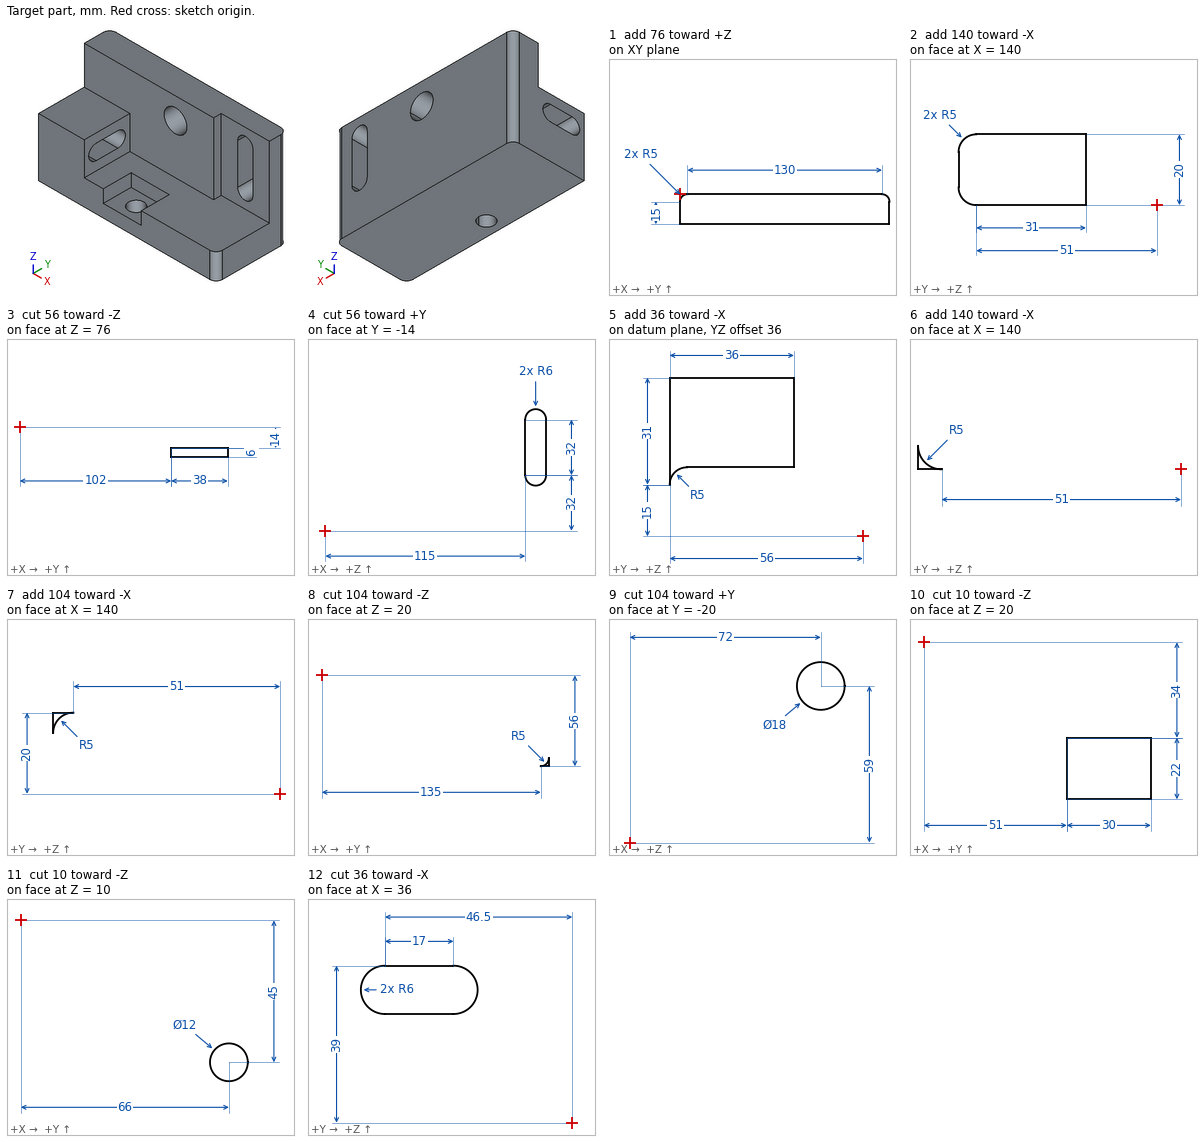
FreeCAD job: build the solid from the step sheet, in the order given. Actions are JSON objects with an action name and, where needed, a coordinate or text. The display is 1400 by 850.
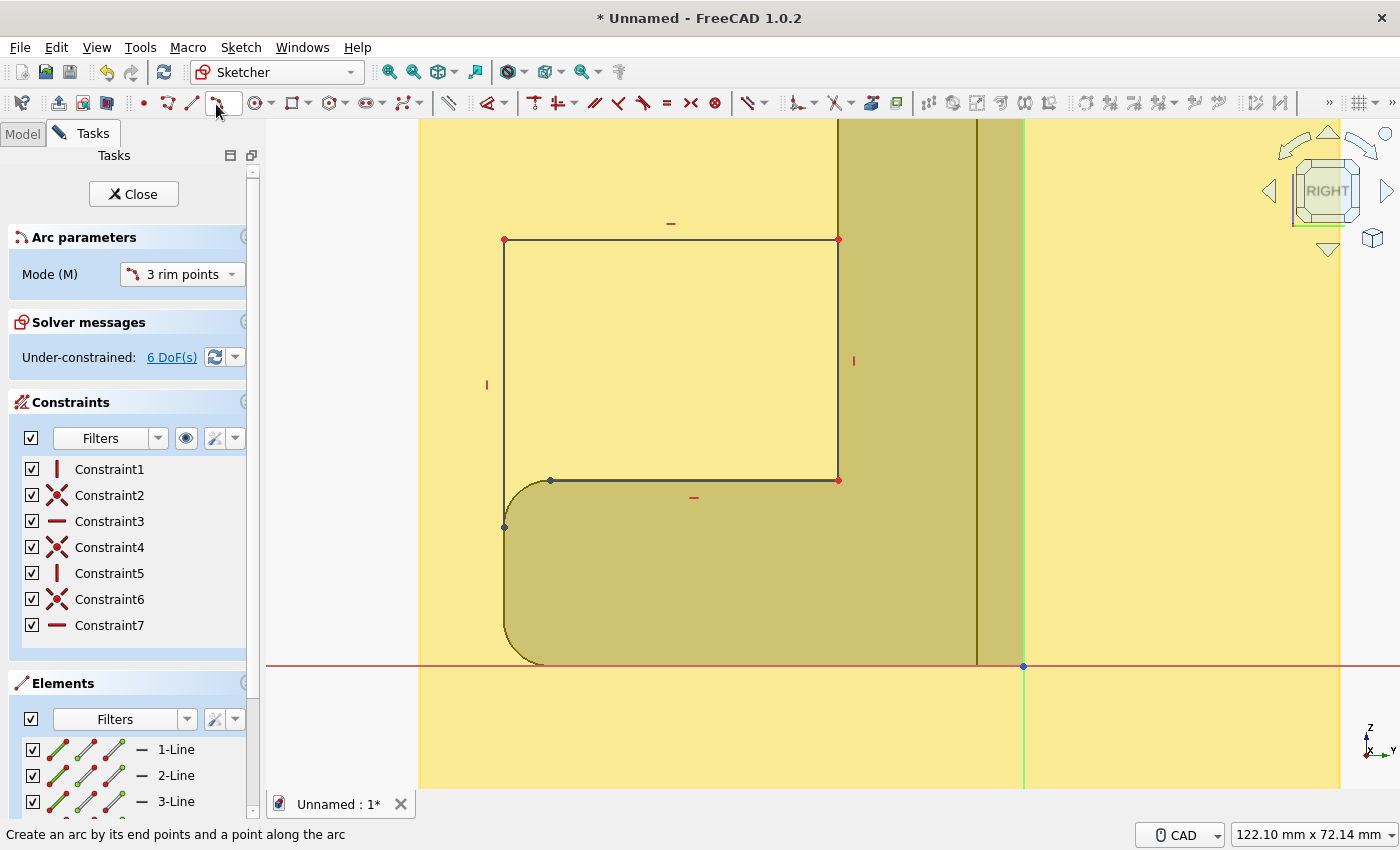
{"action": "left_click", "coordinate": [550, 481]}
{"action": "left_click", "coordinate": [504, 528]}
{"action": "left_click", "coordinate": [517, 494]}
{"action": "key", "text": "Escape"}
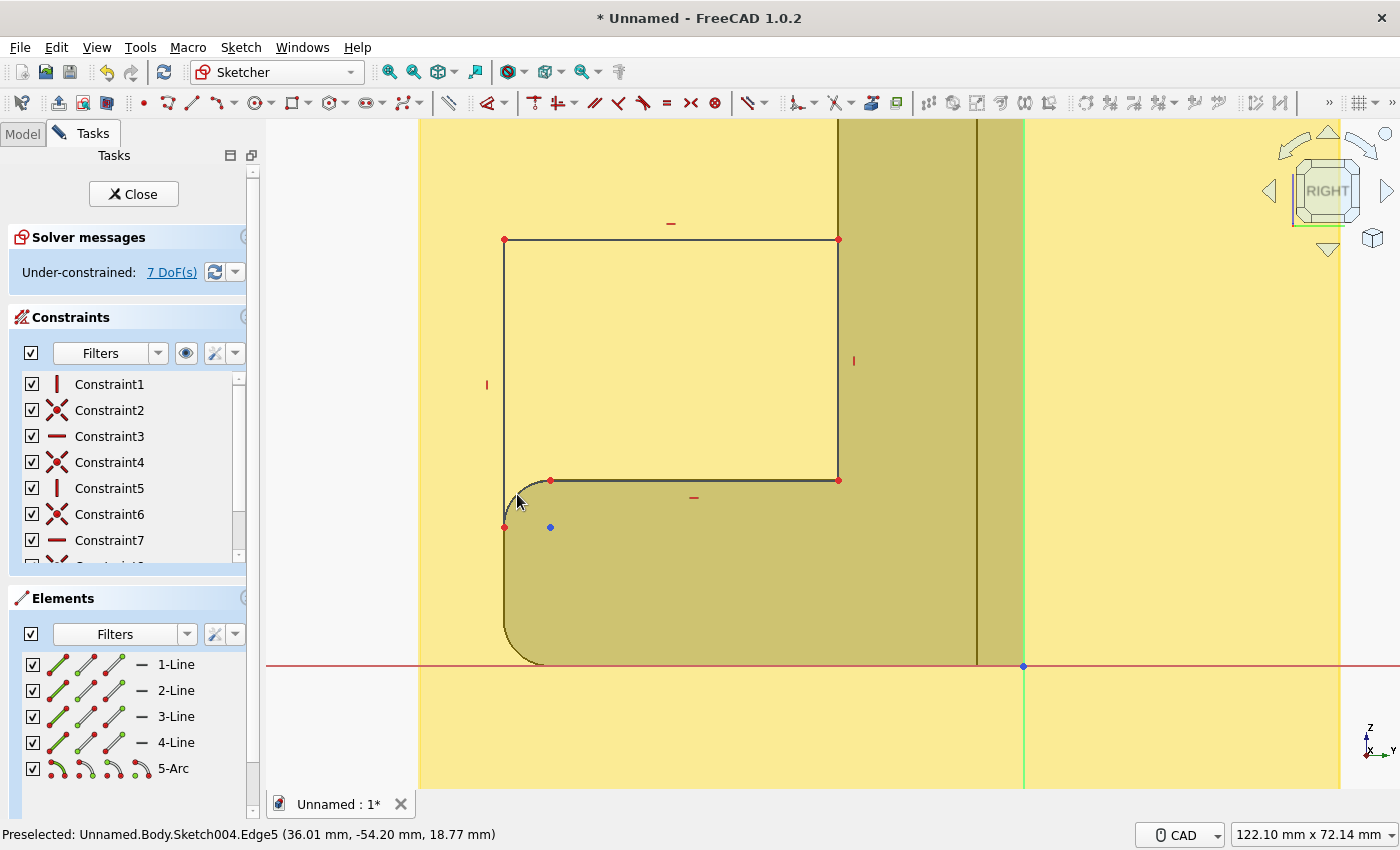
{"action": "left_click", "coordinate": [504, 442]}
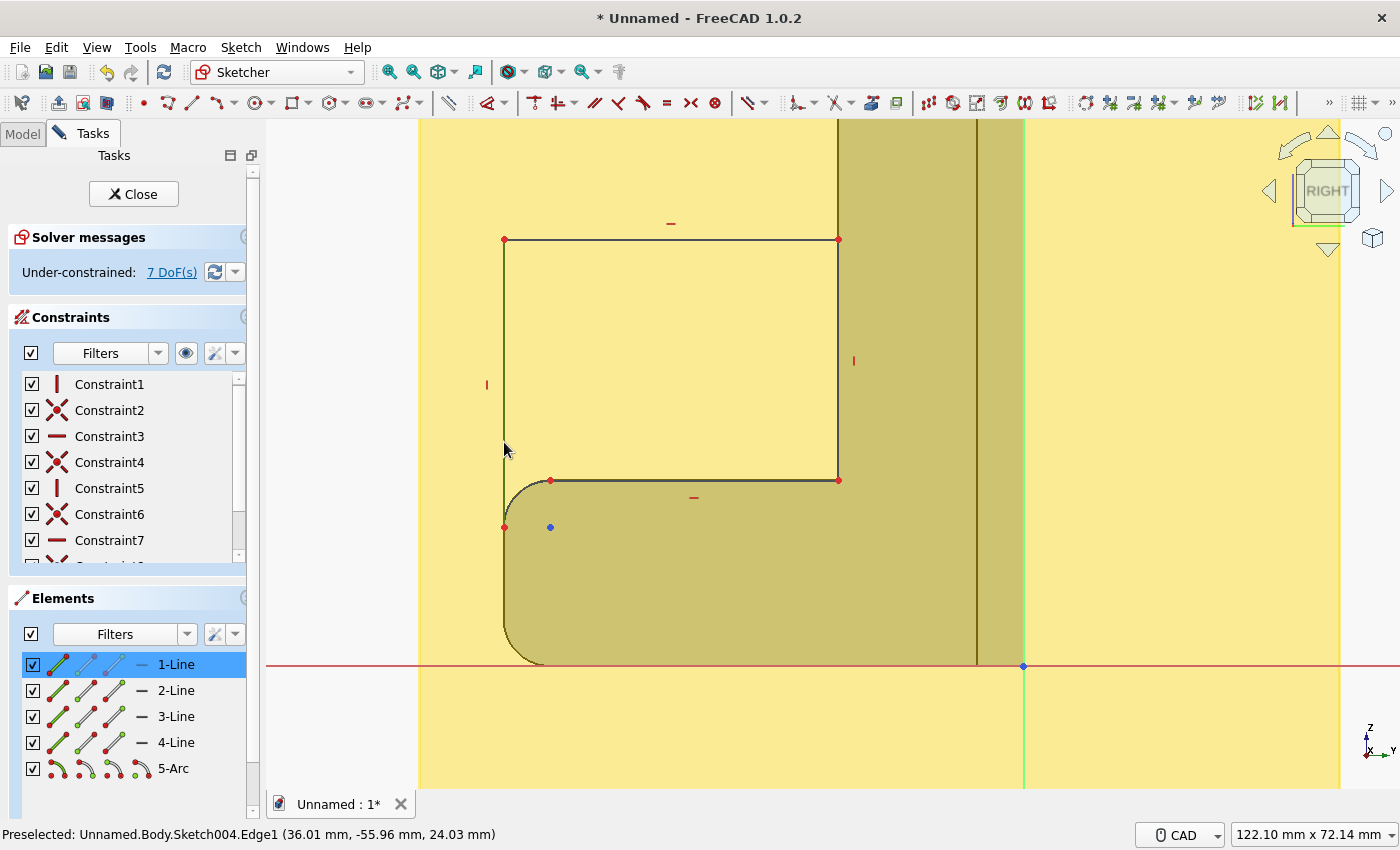
{"action": "left_click", "coordinate": [529, 486]}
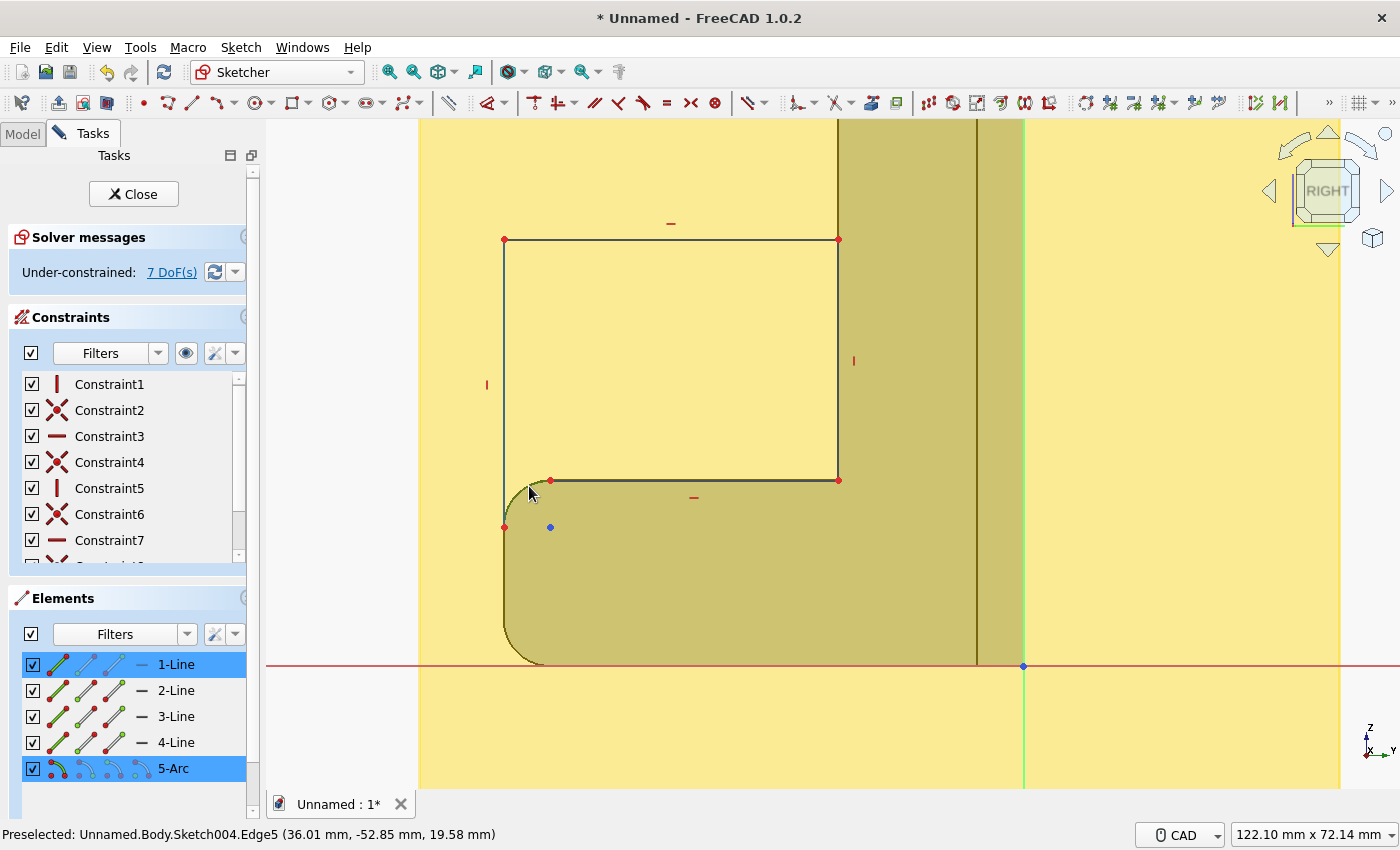
{"action": "left_click", "coordinate": [644, 104]}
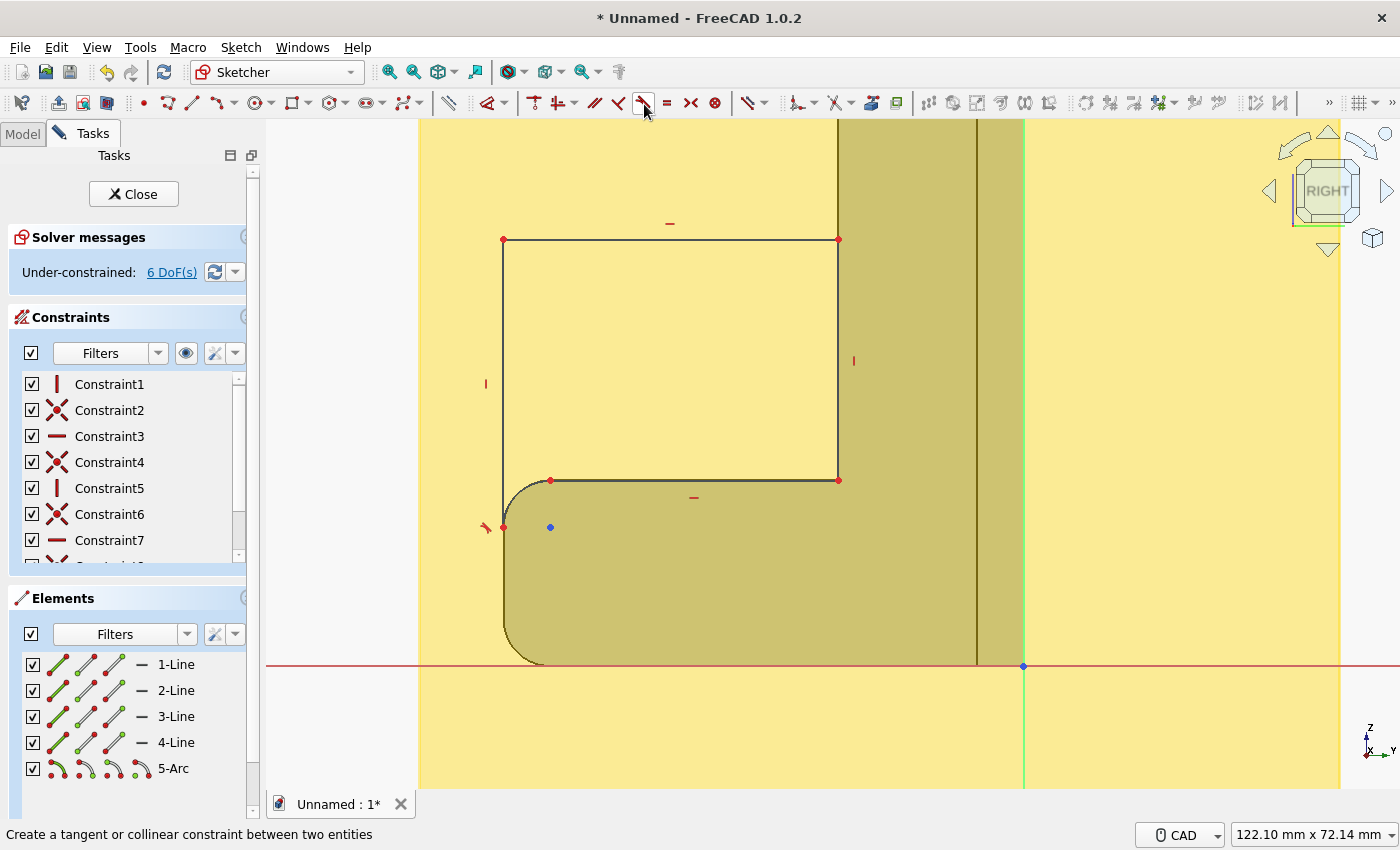
{"action": "left_click", "coordinate": [752, 481]}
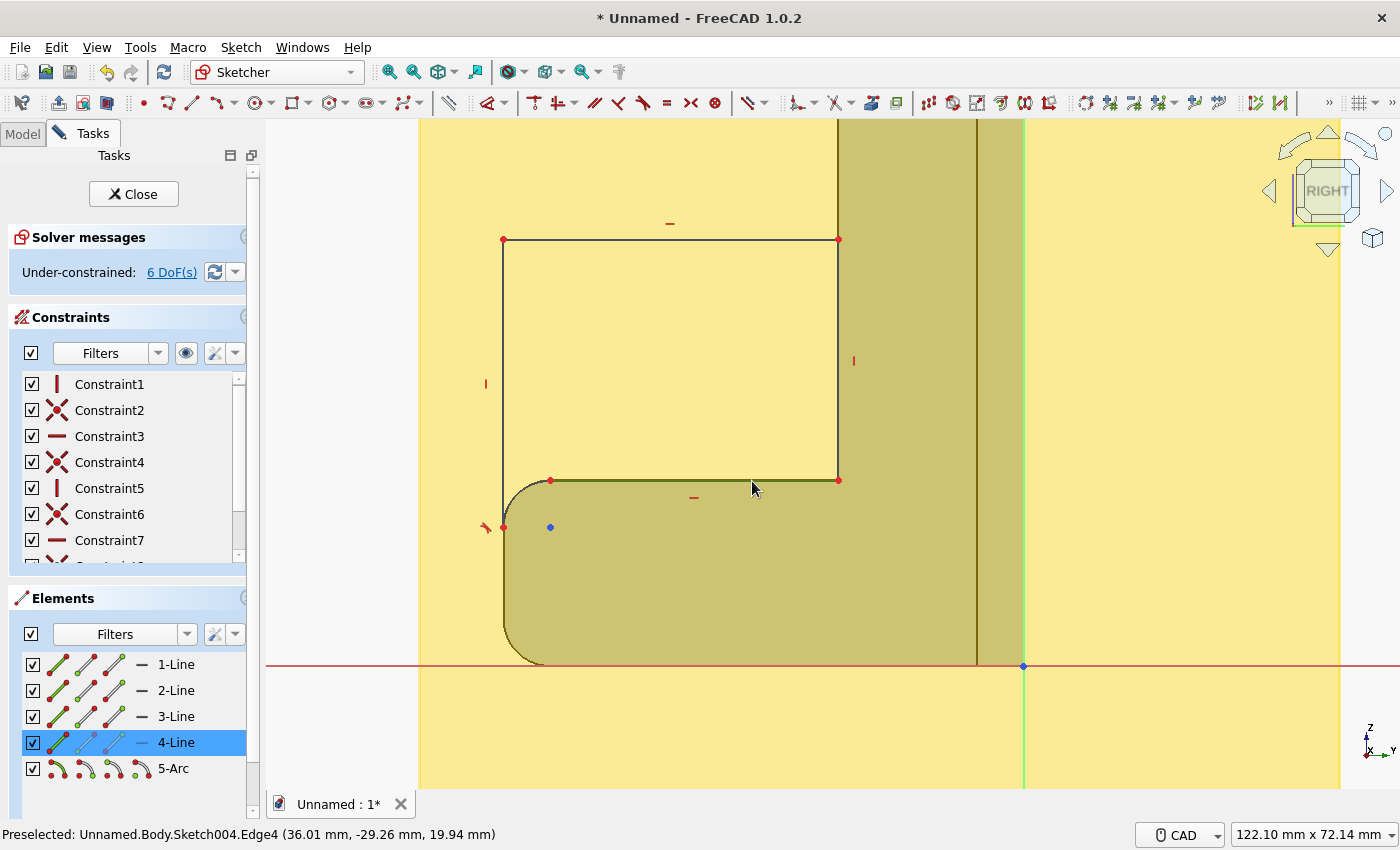
{"action": "left_click", "coordinate": [529, 486]}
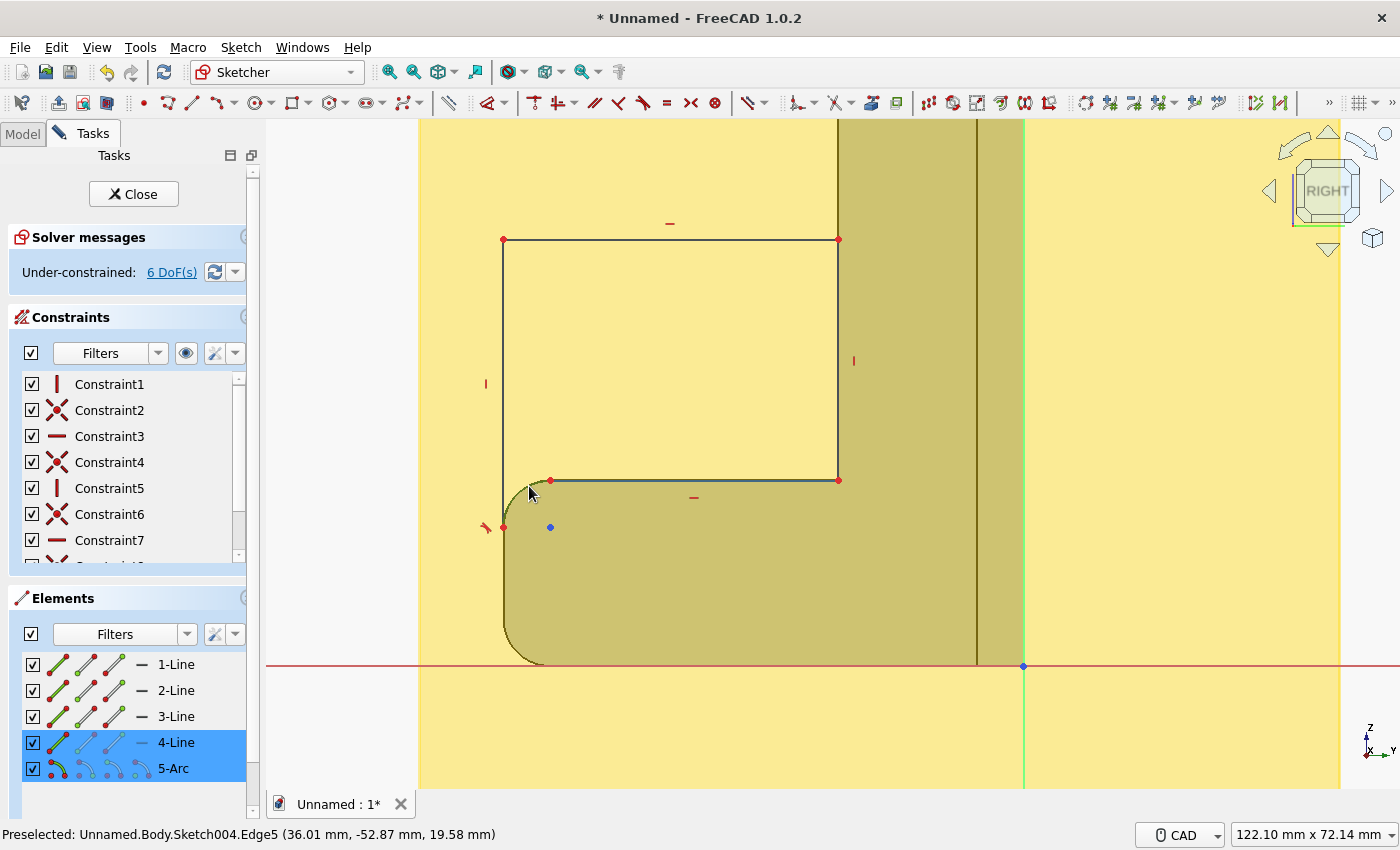
{"action": "left_click", "coordinate": [644, 104]}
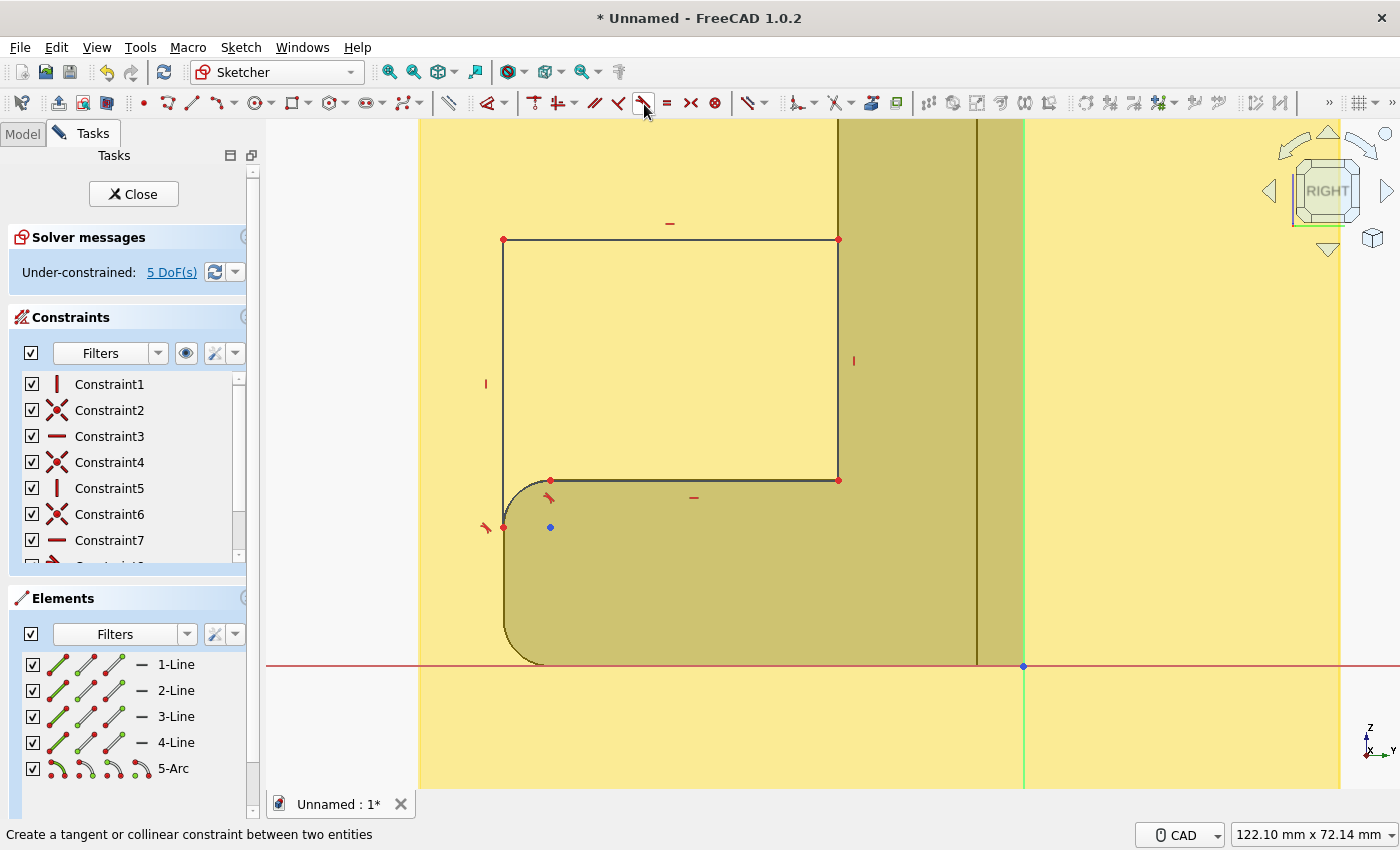
{"action": "left_click", "coordinate": [488, 104]}